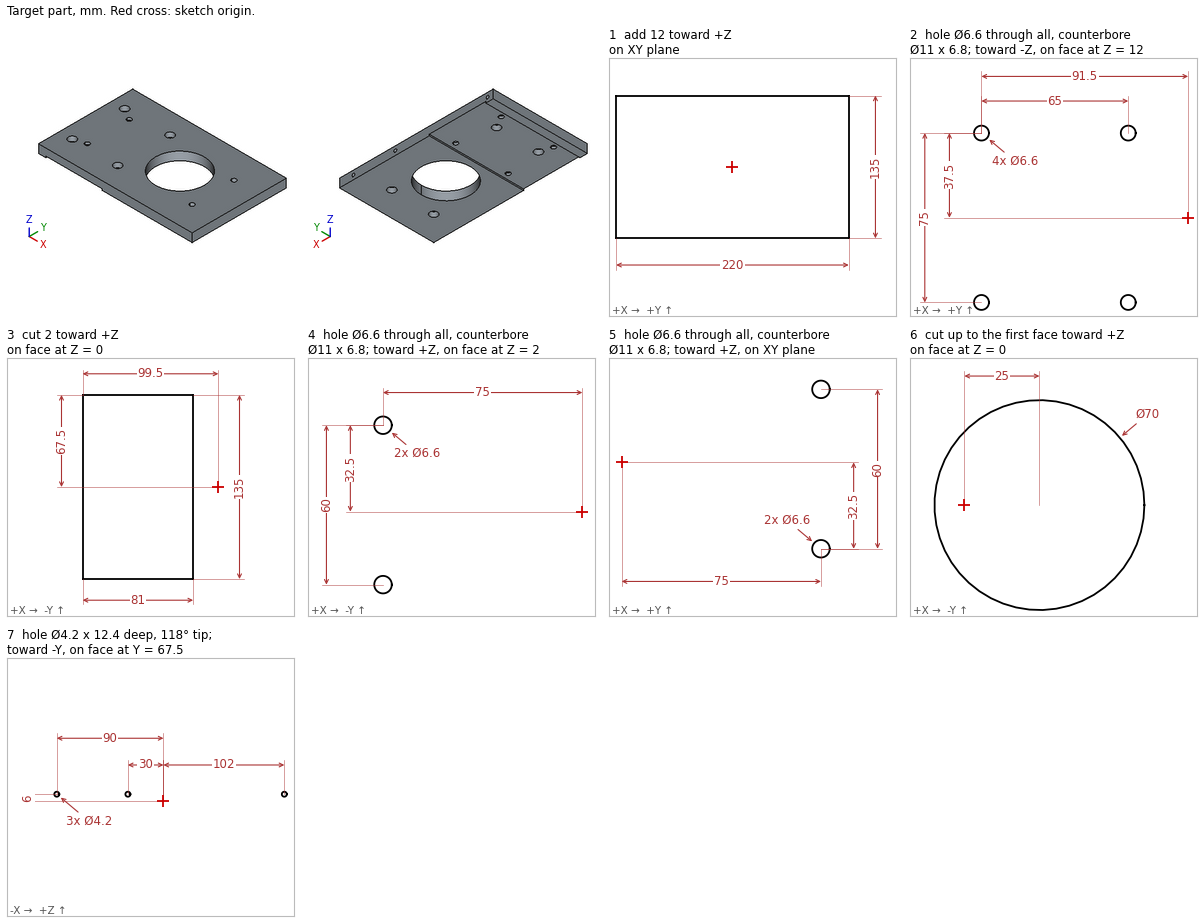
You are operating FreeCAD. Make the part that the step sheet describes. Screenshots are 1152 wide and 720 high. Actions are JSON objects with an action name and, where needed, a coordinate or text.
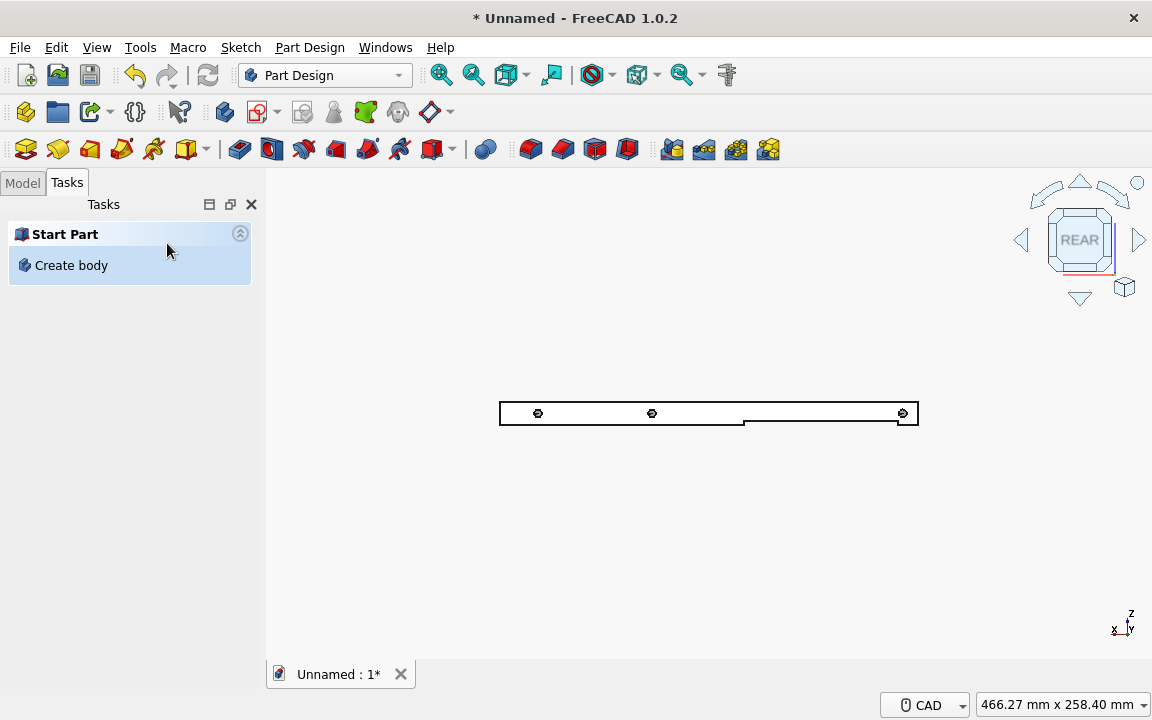
{"action": "key", "text": "0"}